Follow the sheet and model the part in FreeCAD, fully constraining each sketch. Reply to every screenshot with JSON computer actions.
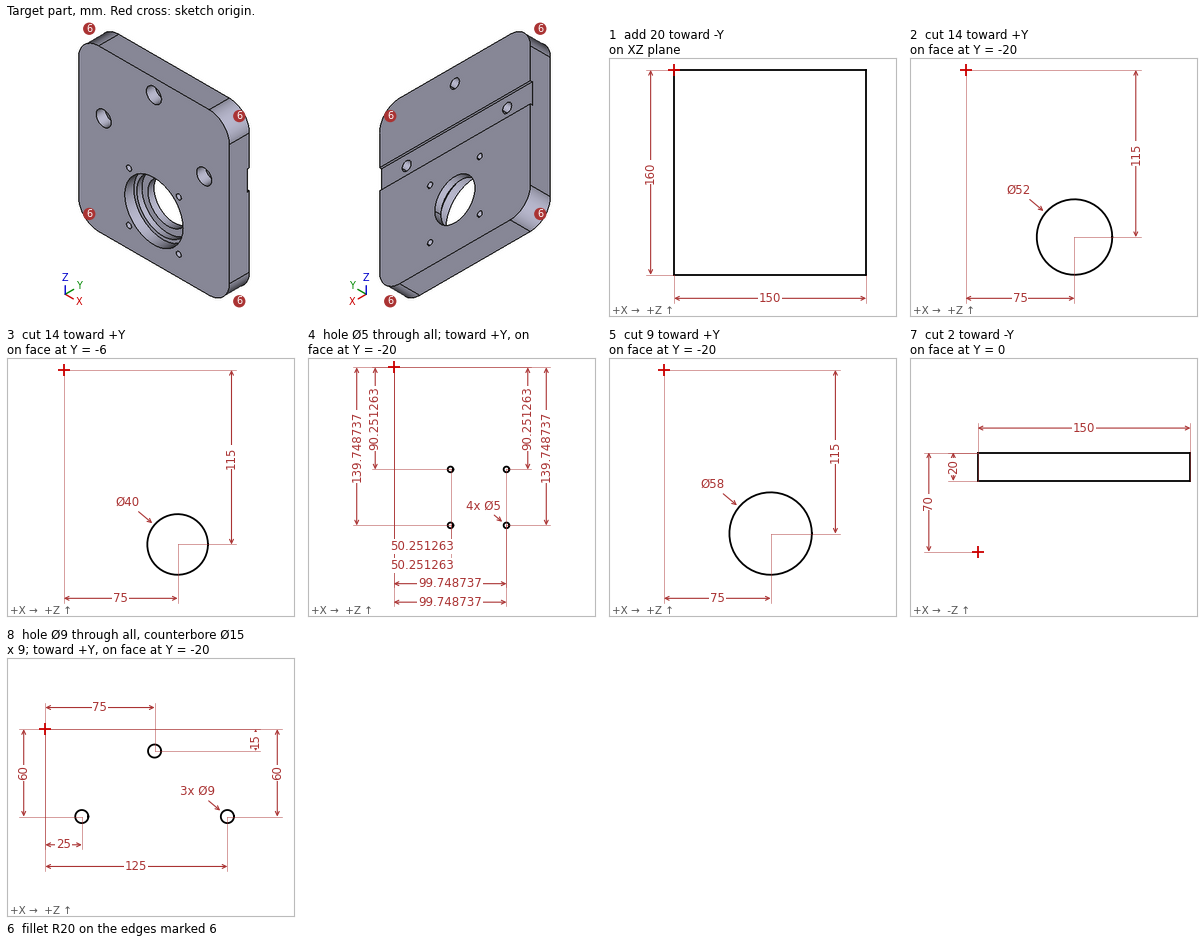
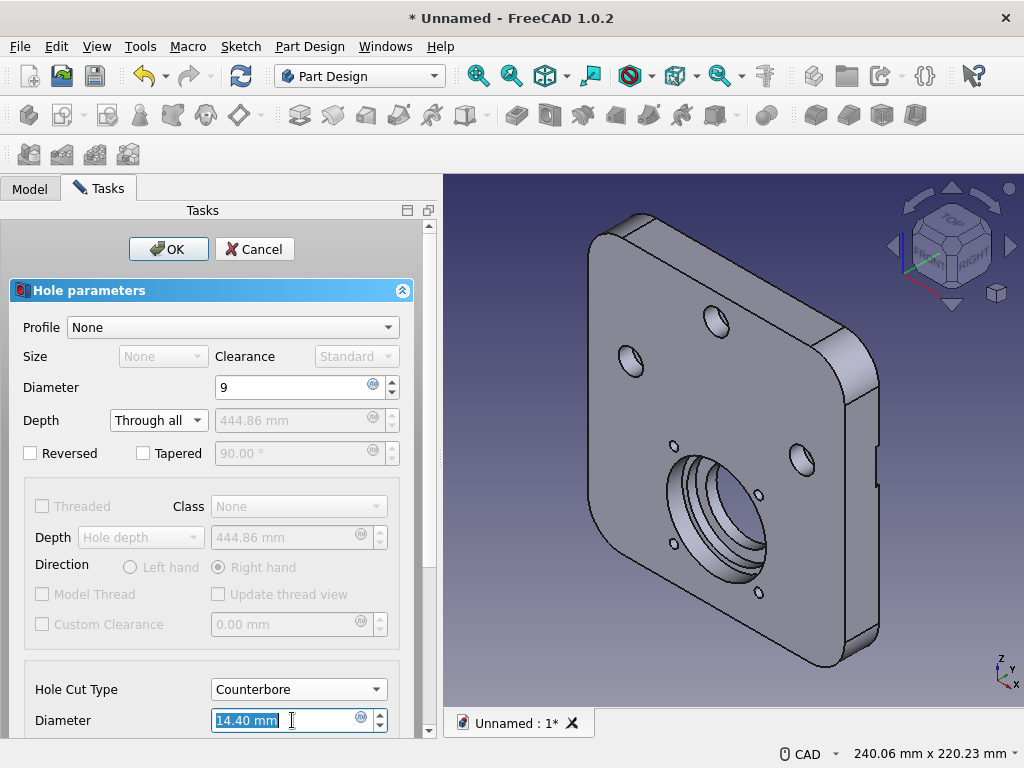
{"action": "type", "text": "15"}
{"action": "key", "text": "Tab"}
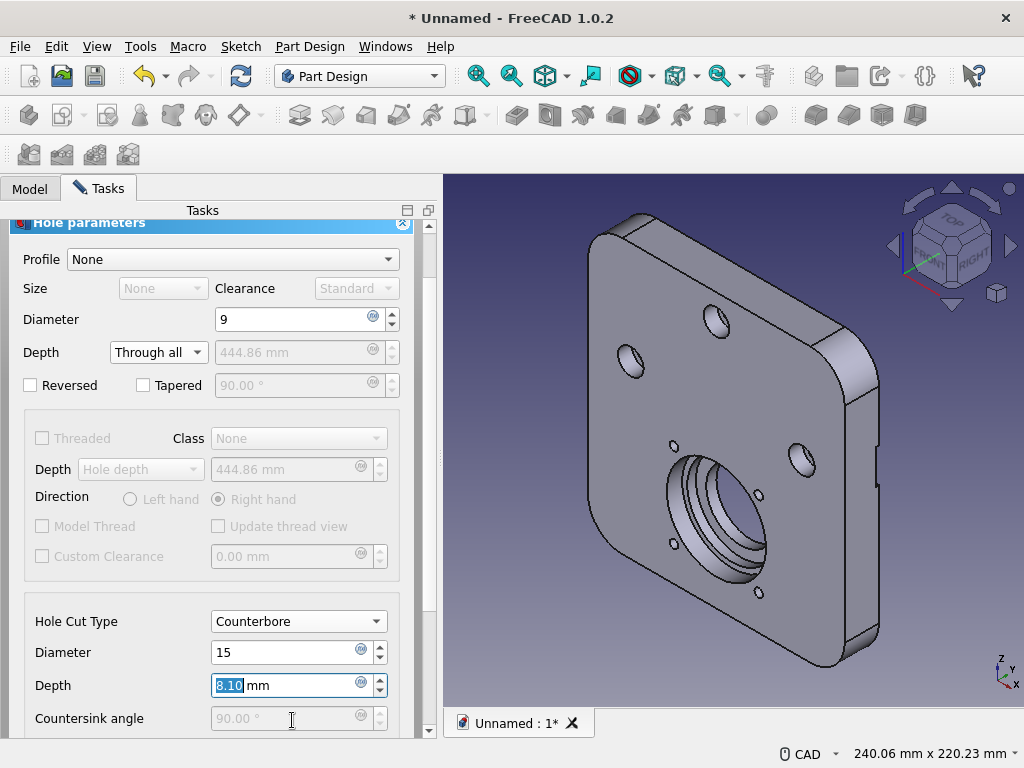
{"action": "type", "text": "9"}
{"action": "key", "text": "Tab"}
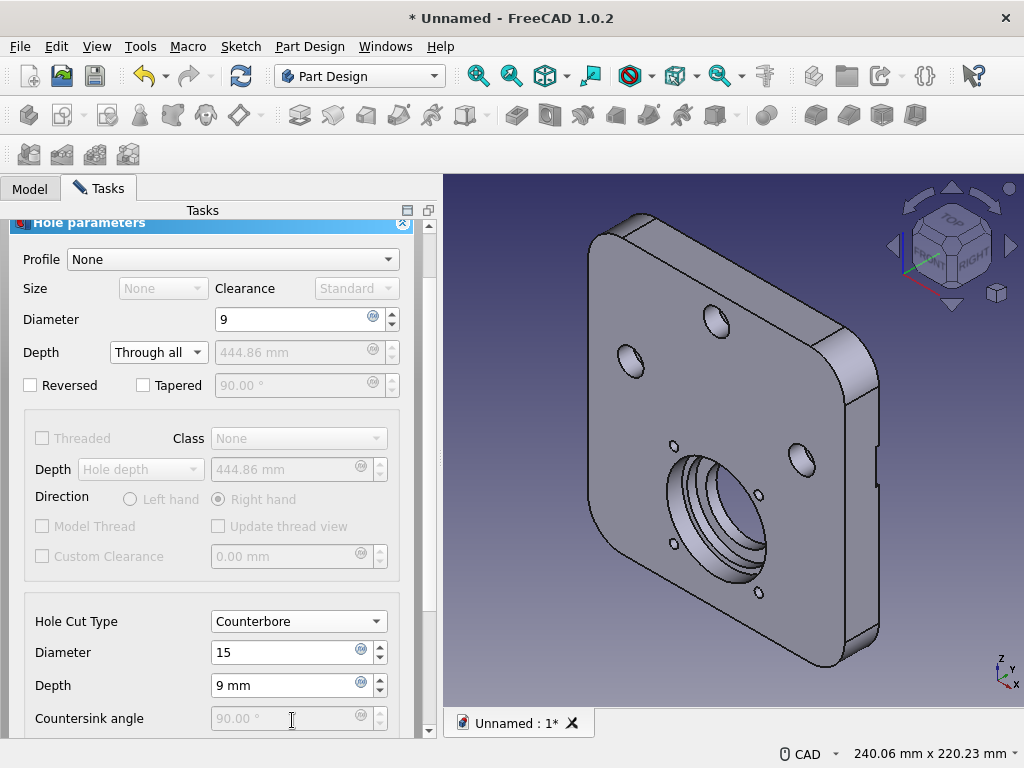
{"action": "scroll", "coordinate": [429, 479], "scroll_direction": "up", "scroll_amount": 2}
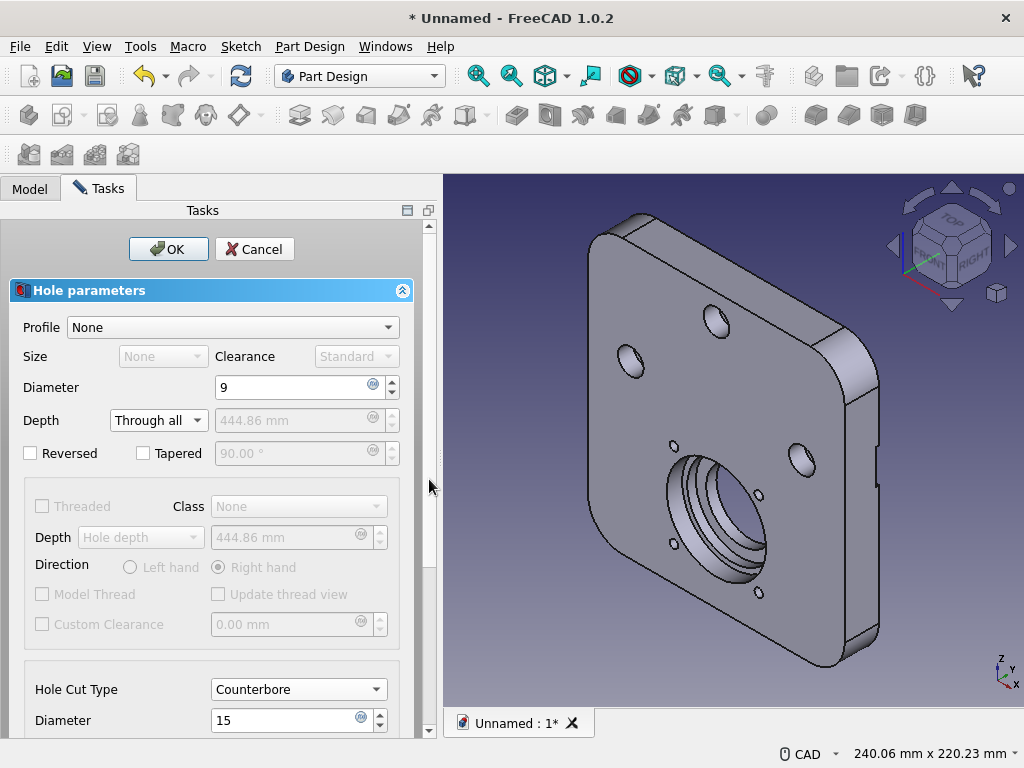
{"action": "left_click", "coordinate": [169, 249]}